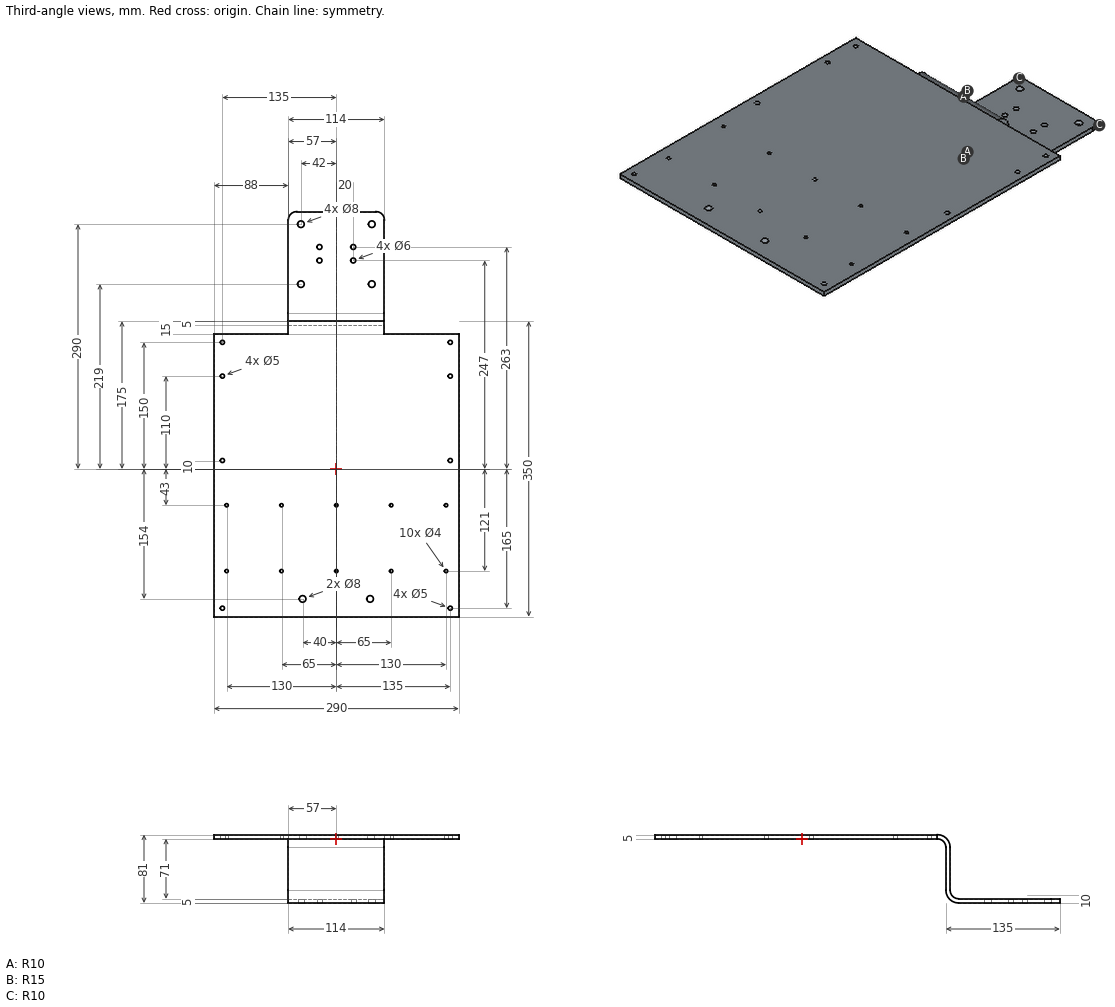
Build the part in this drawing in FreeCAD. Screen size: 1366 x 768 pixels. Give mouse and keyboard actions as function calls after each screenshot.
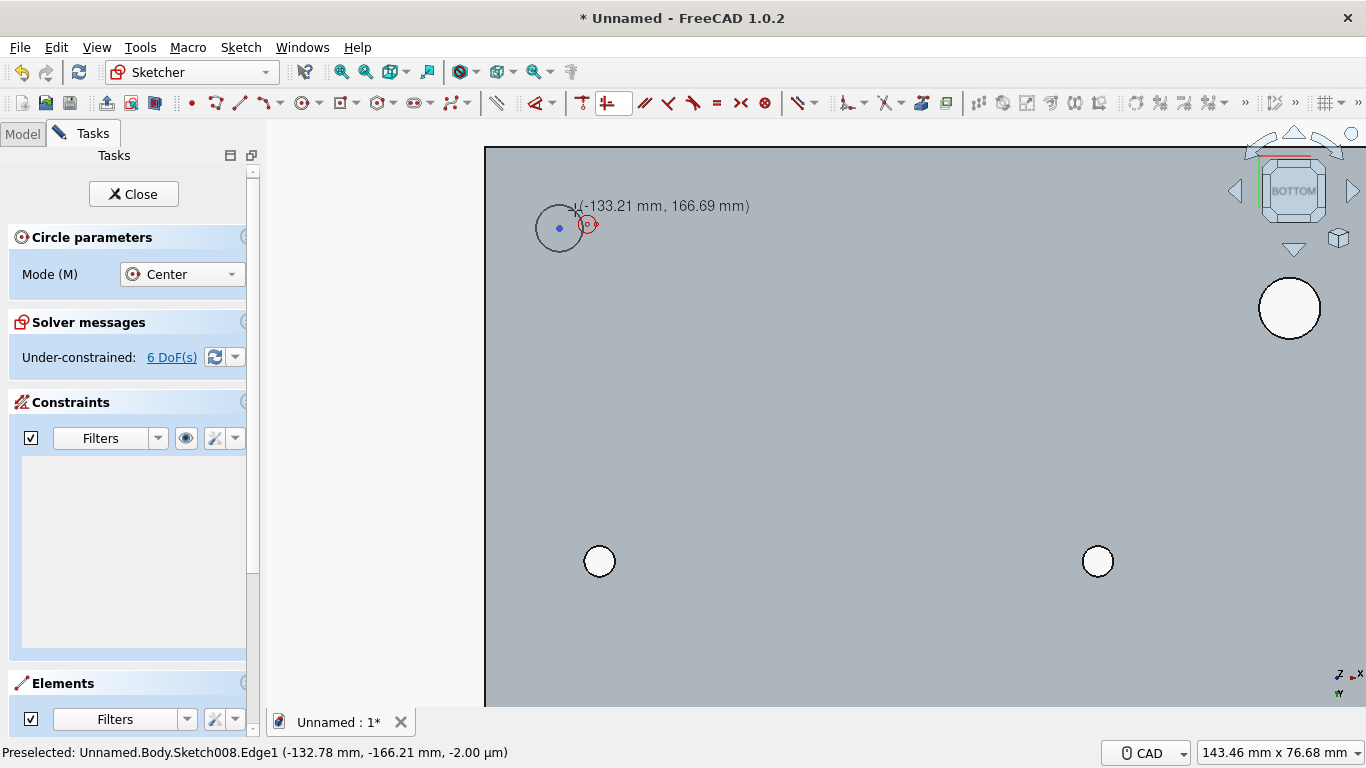
scroll(579, 211, down, 9)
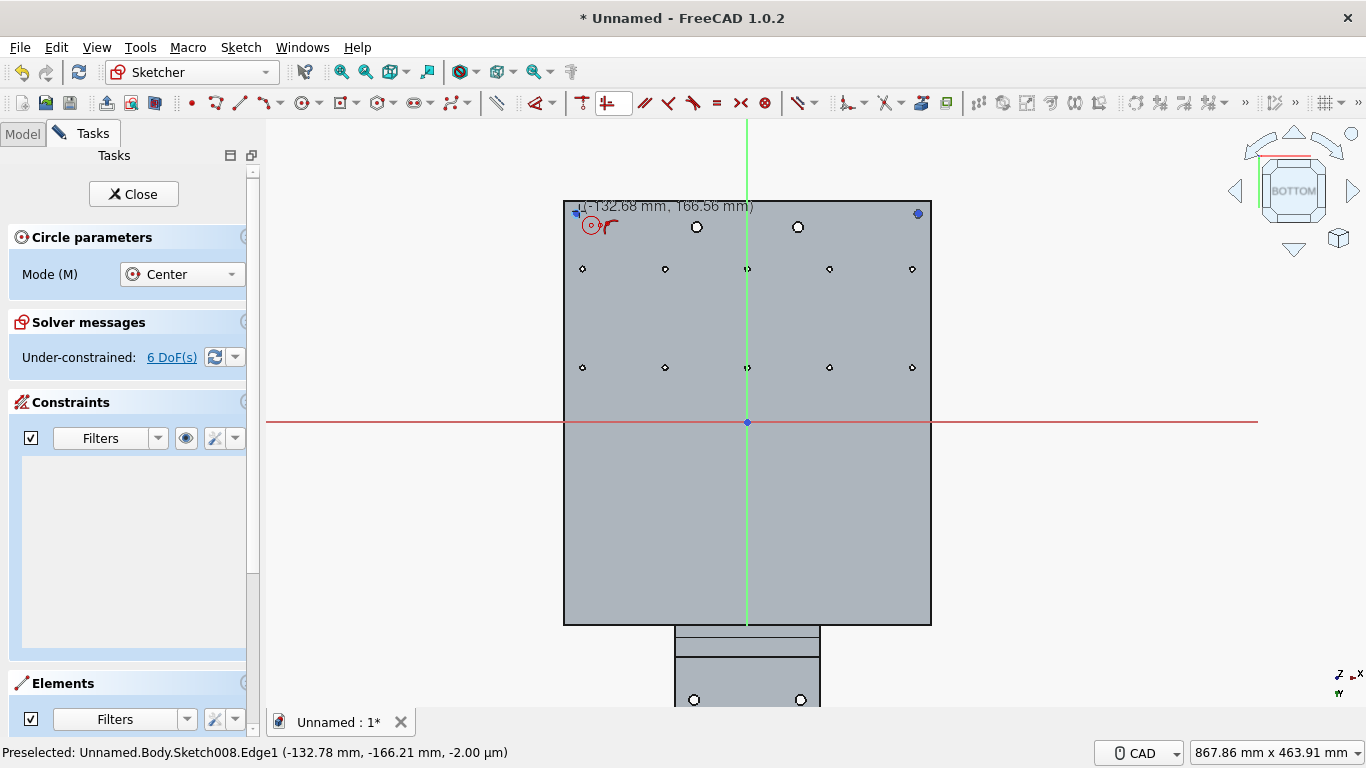
scroll(576, 613, up, 10)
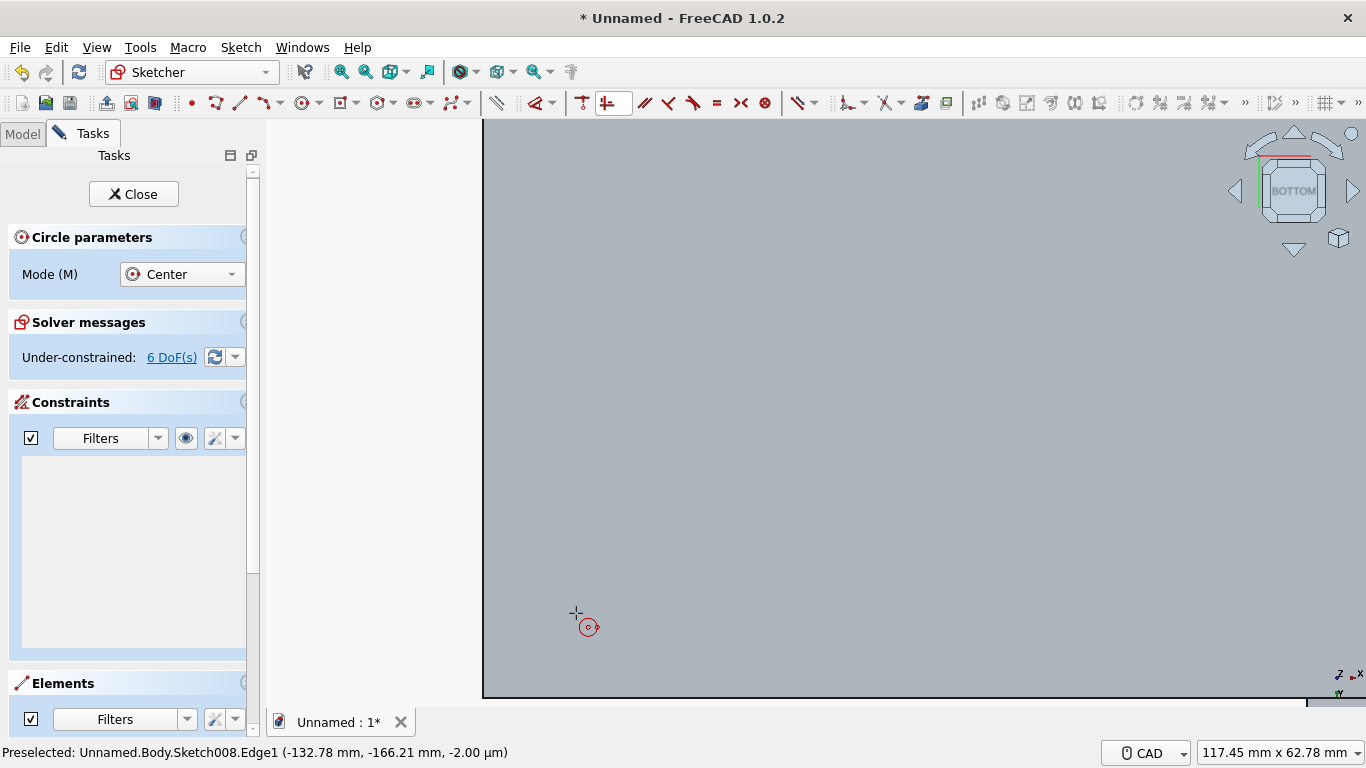
scroll(576, 614, down, 10)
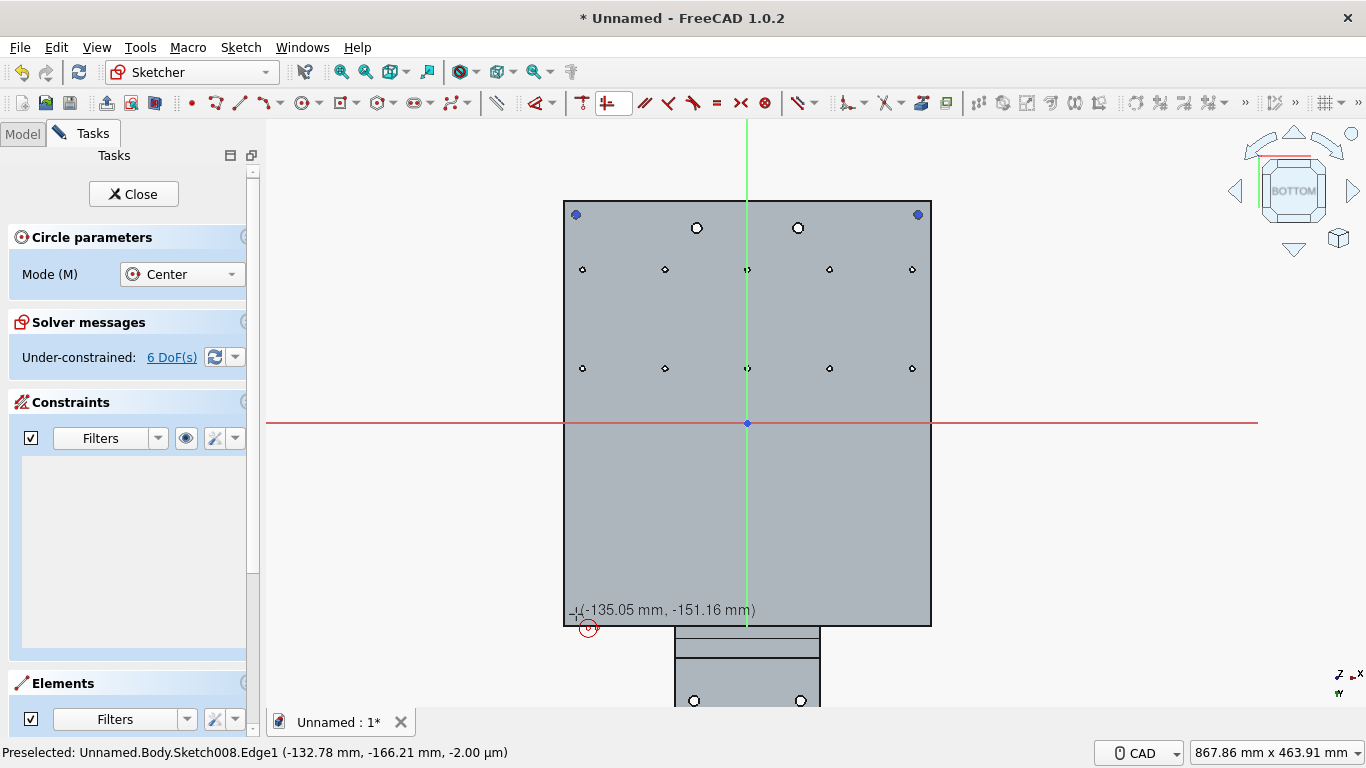
click(576, 613)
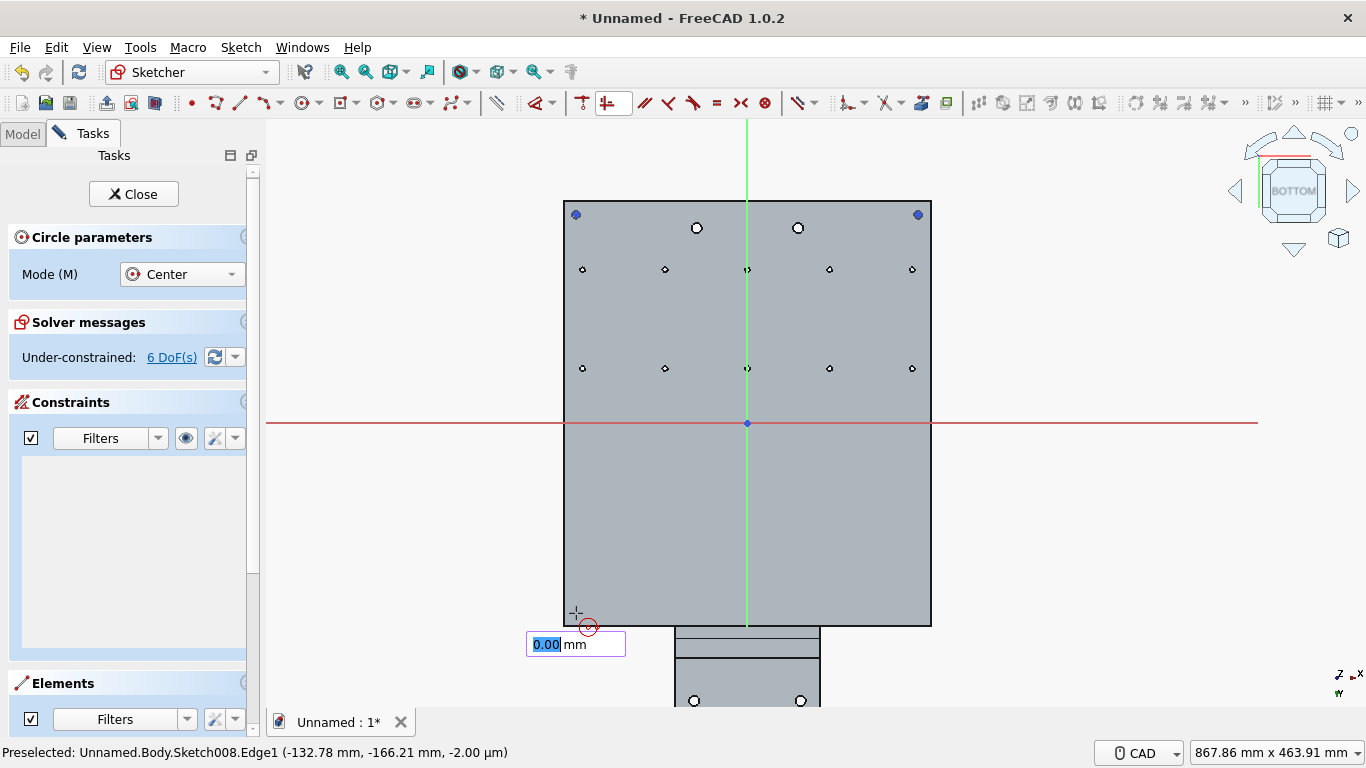
scroll(579, 611, up, 9)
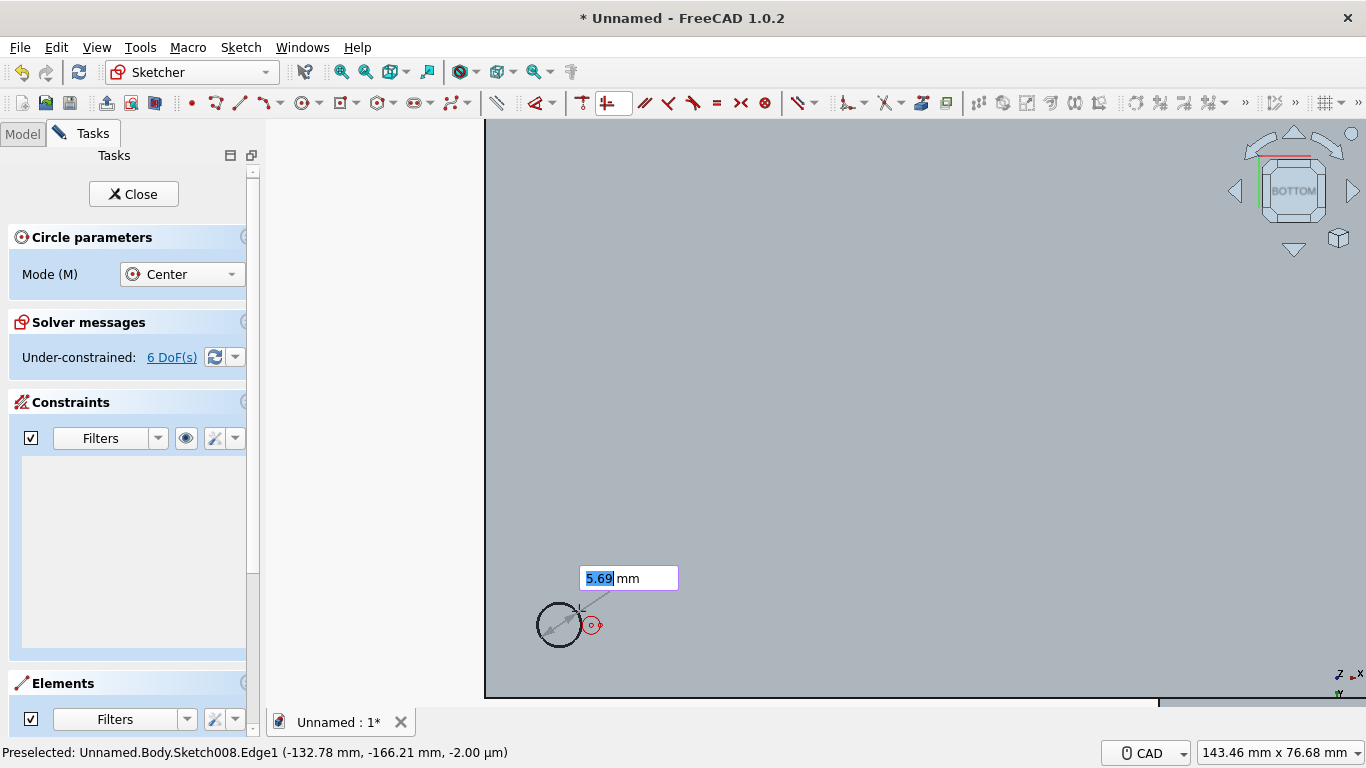
click(575, 608)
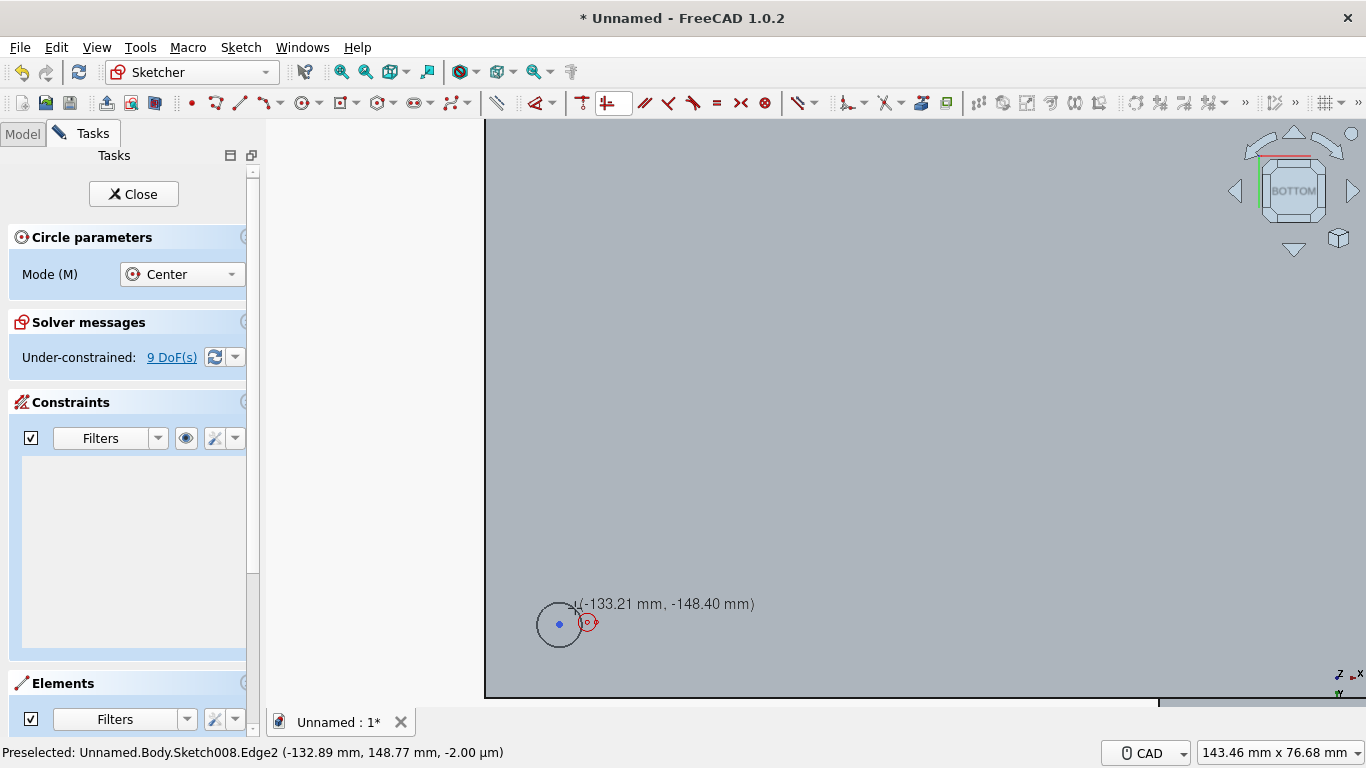
scroll(579, 611, down, 9)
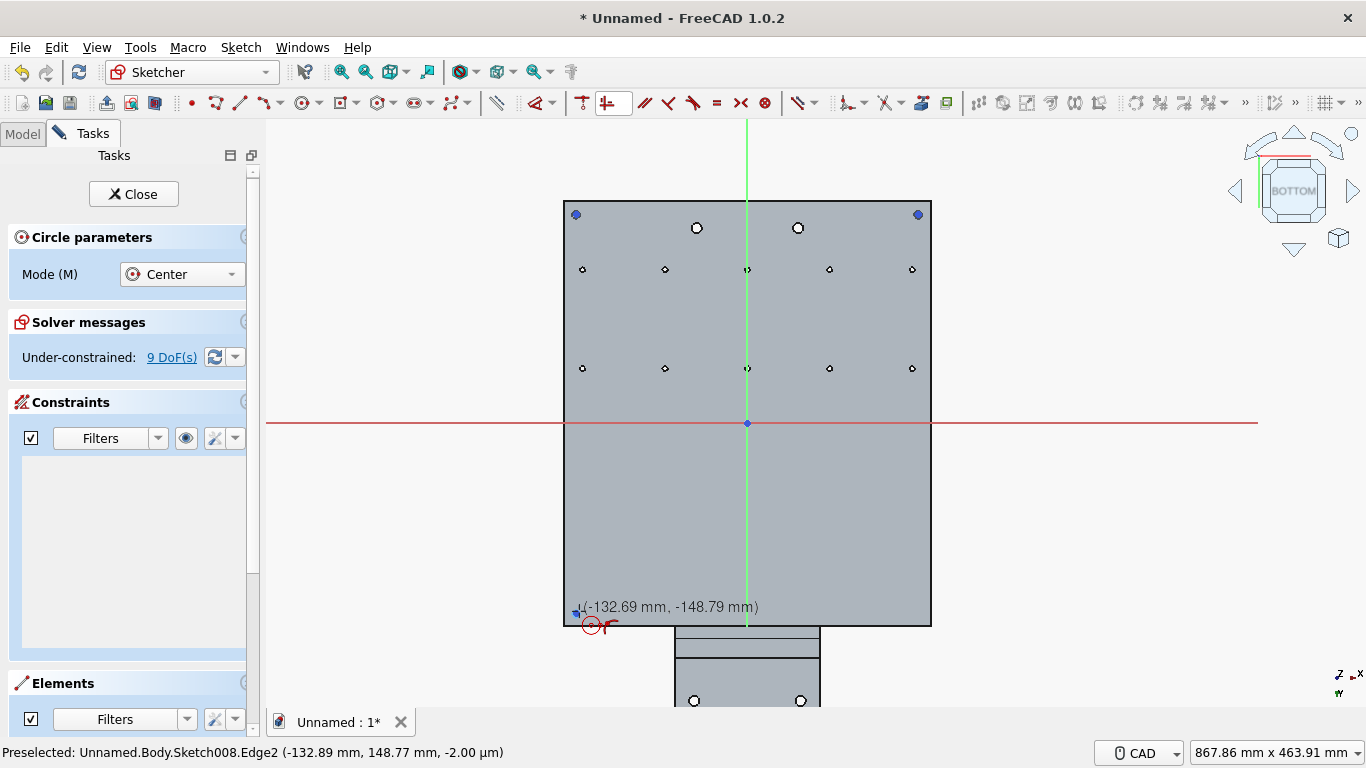
scroll(919, 613, up, 10)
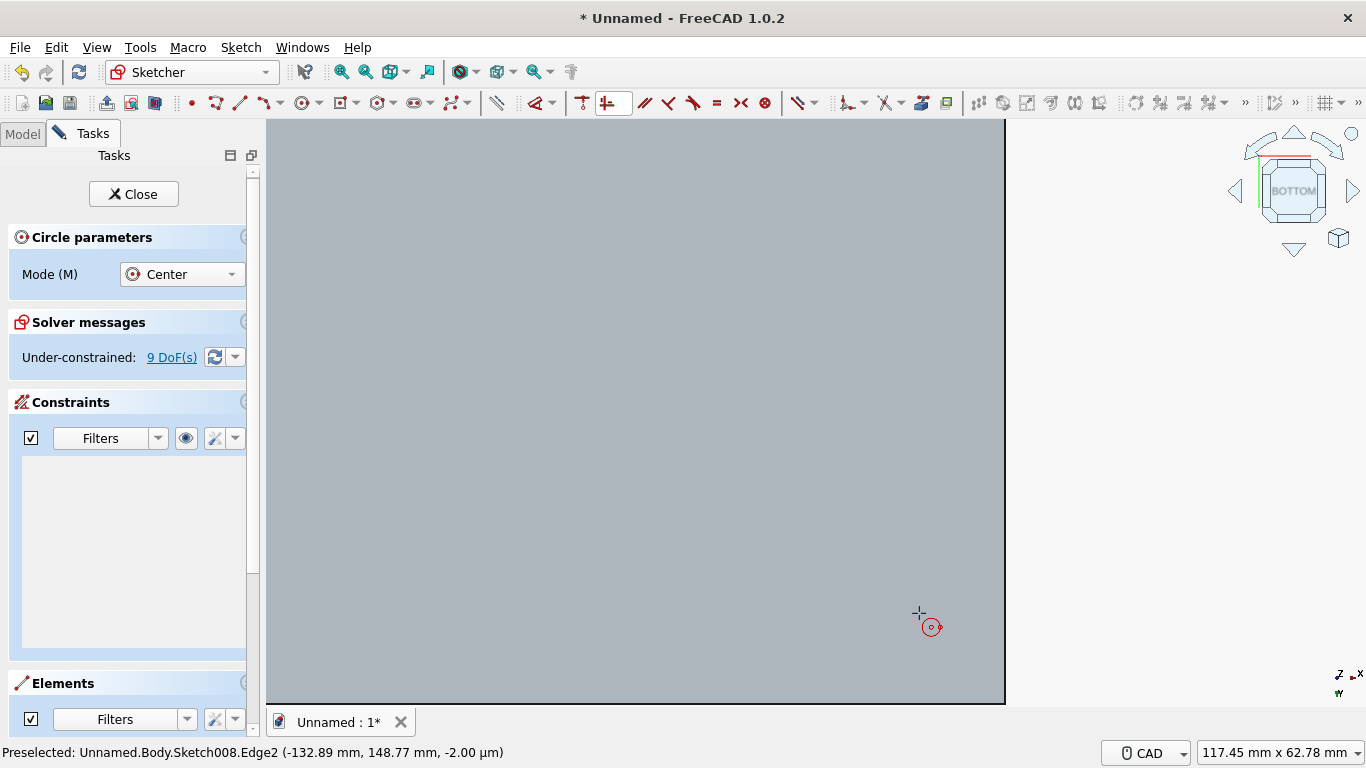
scroll(920, 613, down, 10)